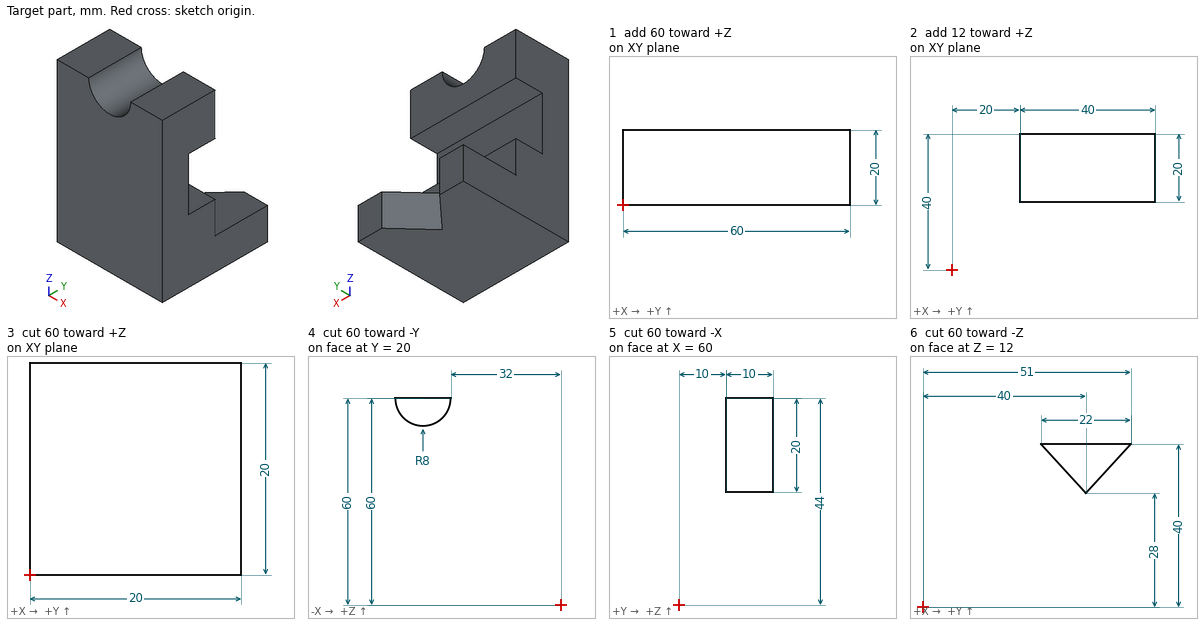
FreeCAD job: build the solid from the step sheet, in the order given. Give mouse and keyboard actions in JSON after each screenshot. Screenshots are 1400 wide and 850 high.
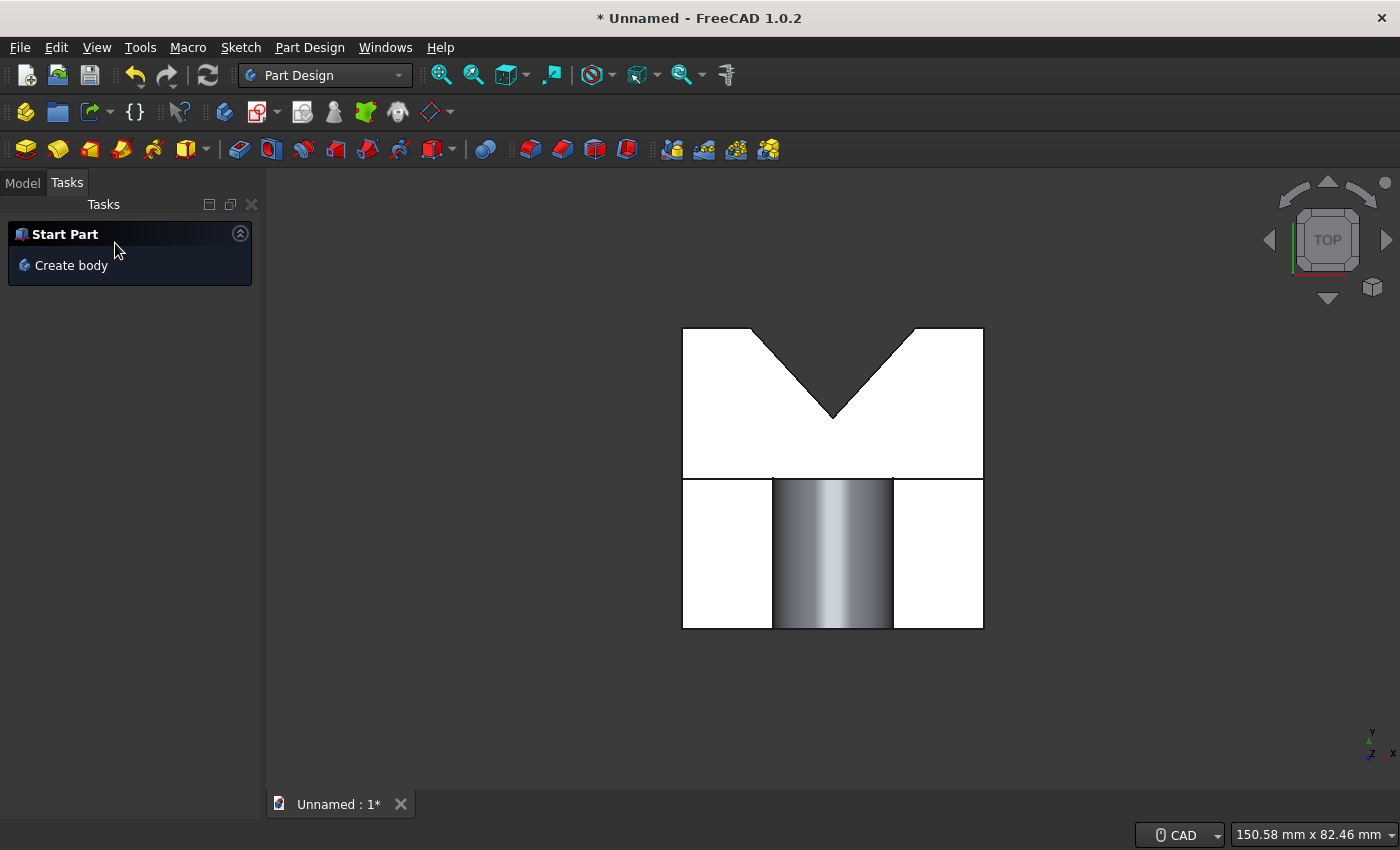
{"action": "key", "text": "0"}